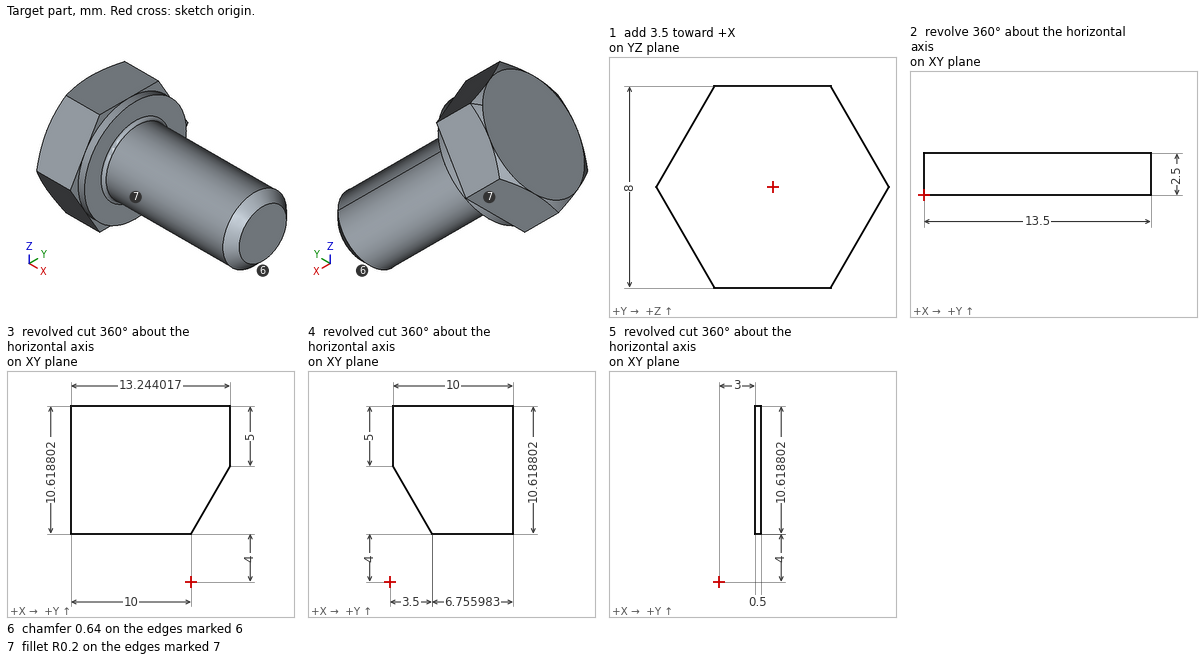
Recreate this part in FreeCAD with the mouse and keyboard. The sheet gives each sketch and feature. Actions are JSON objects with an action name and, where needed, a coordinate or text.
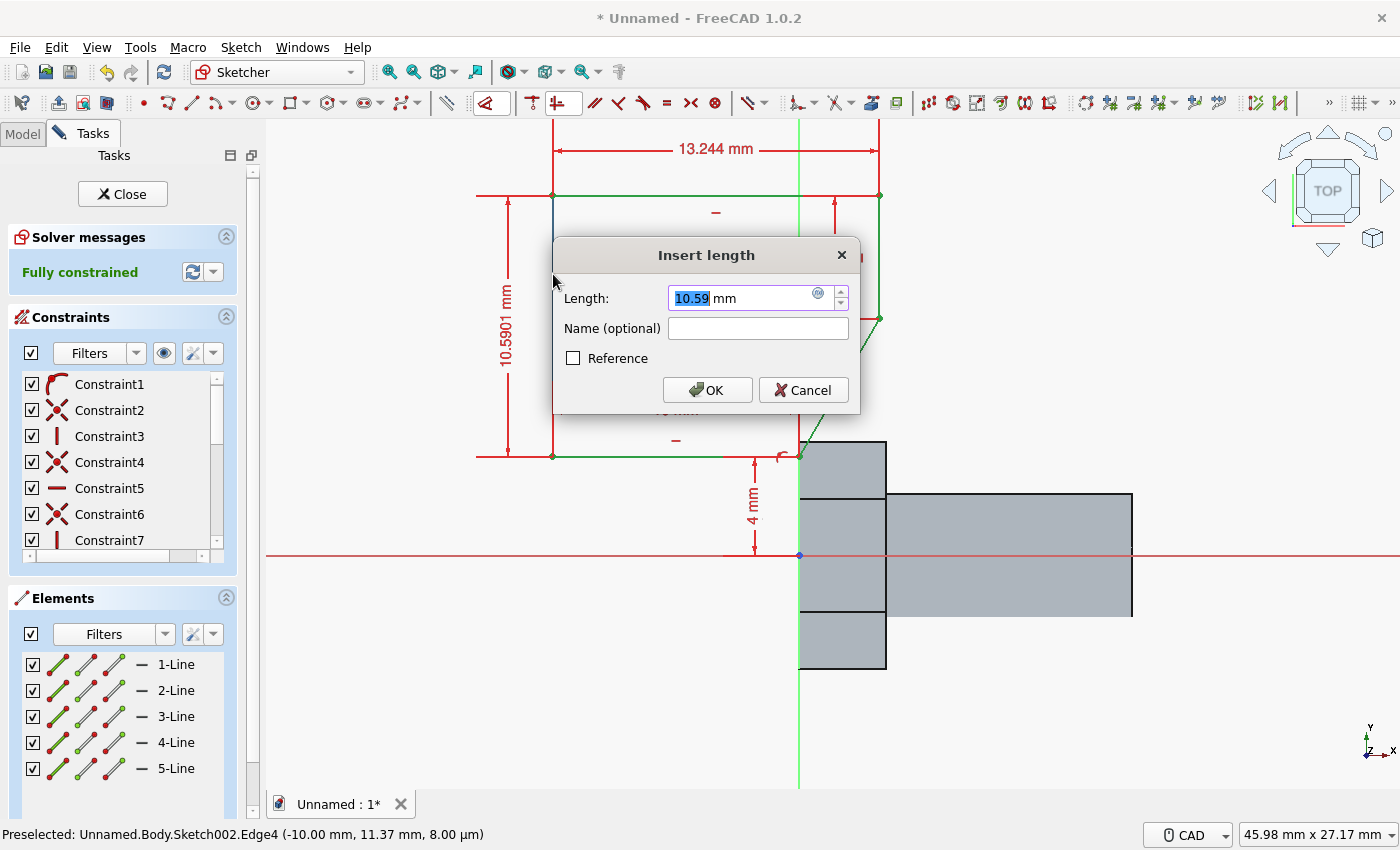
{"action": "type", "text": "10.618802"}
{"action": "key", "text": "Return"}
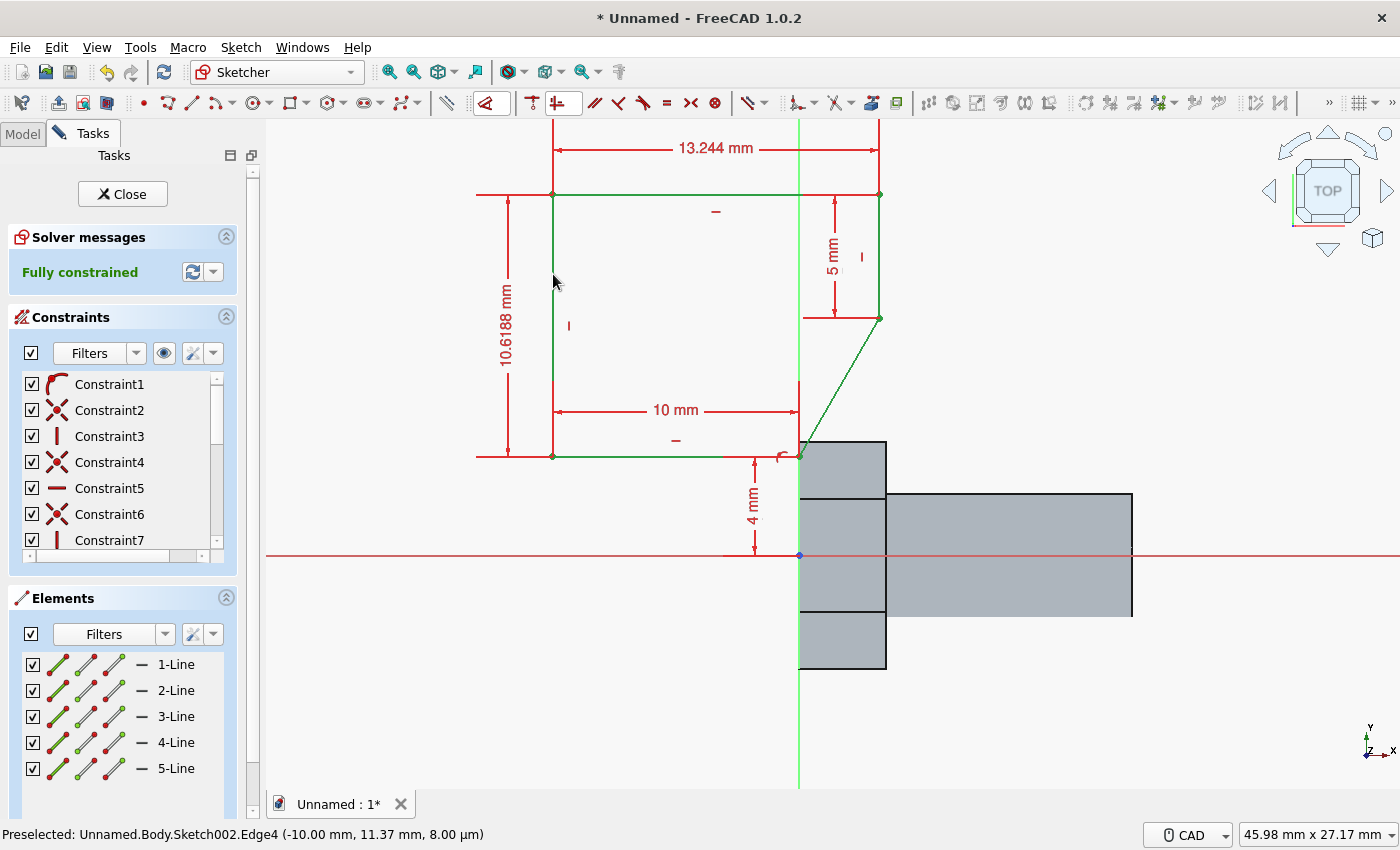
{"action": "left_click", "coordinate": [123, 194]}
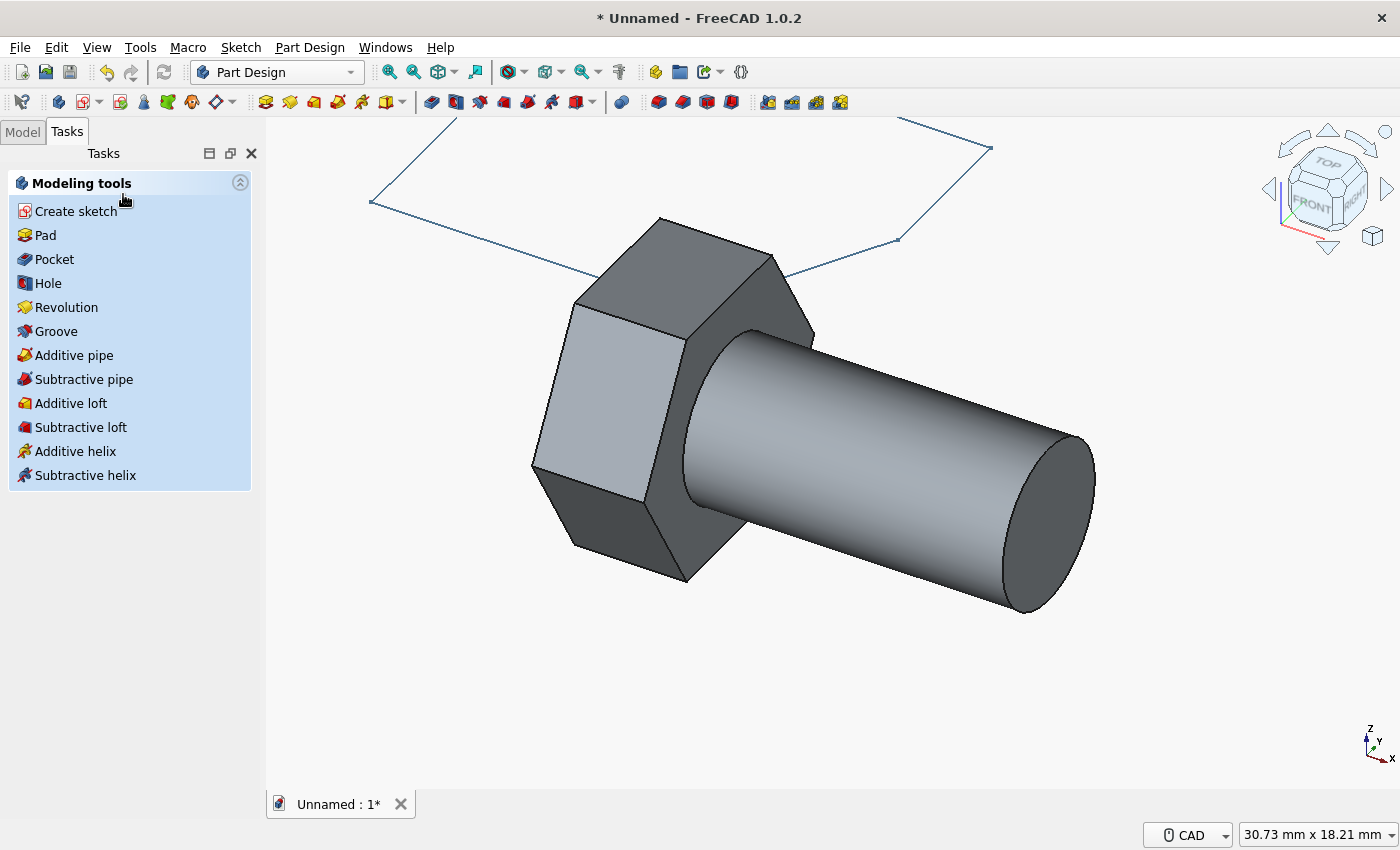
{"action": "left_click", "coordinate": [480, 102]}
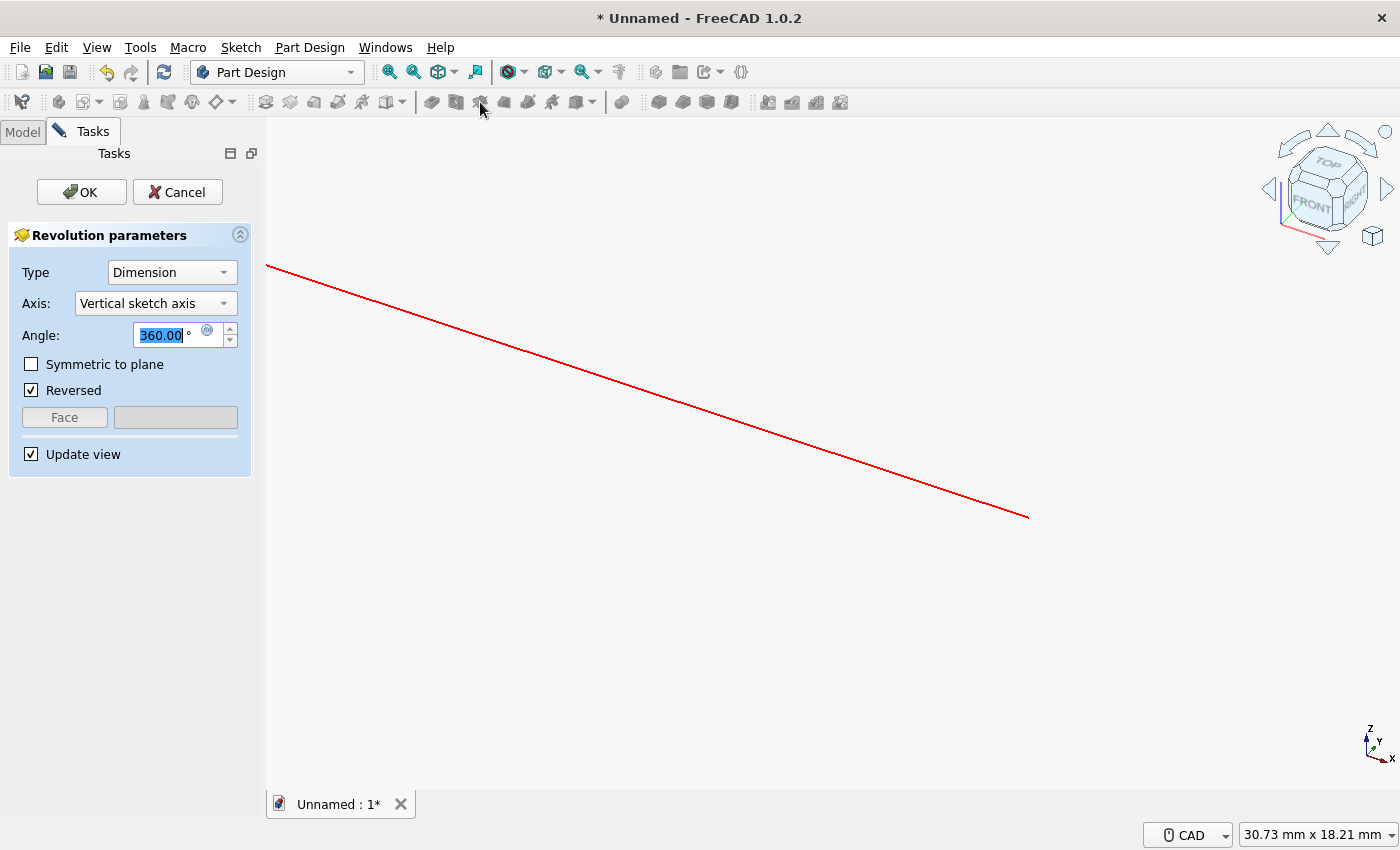
{"action": "left_click", "coordinate": [156, 304]}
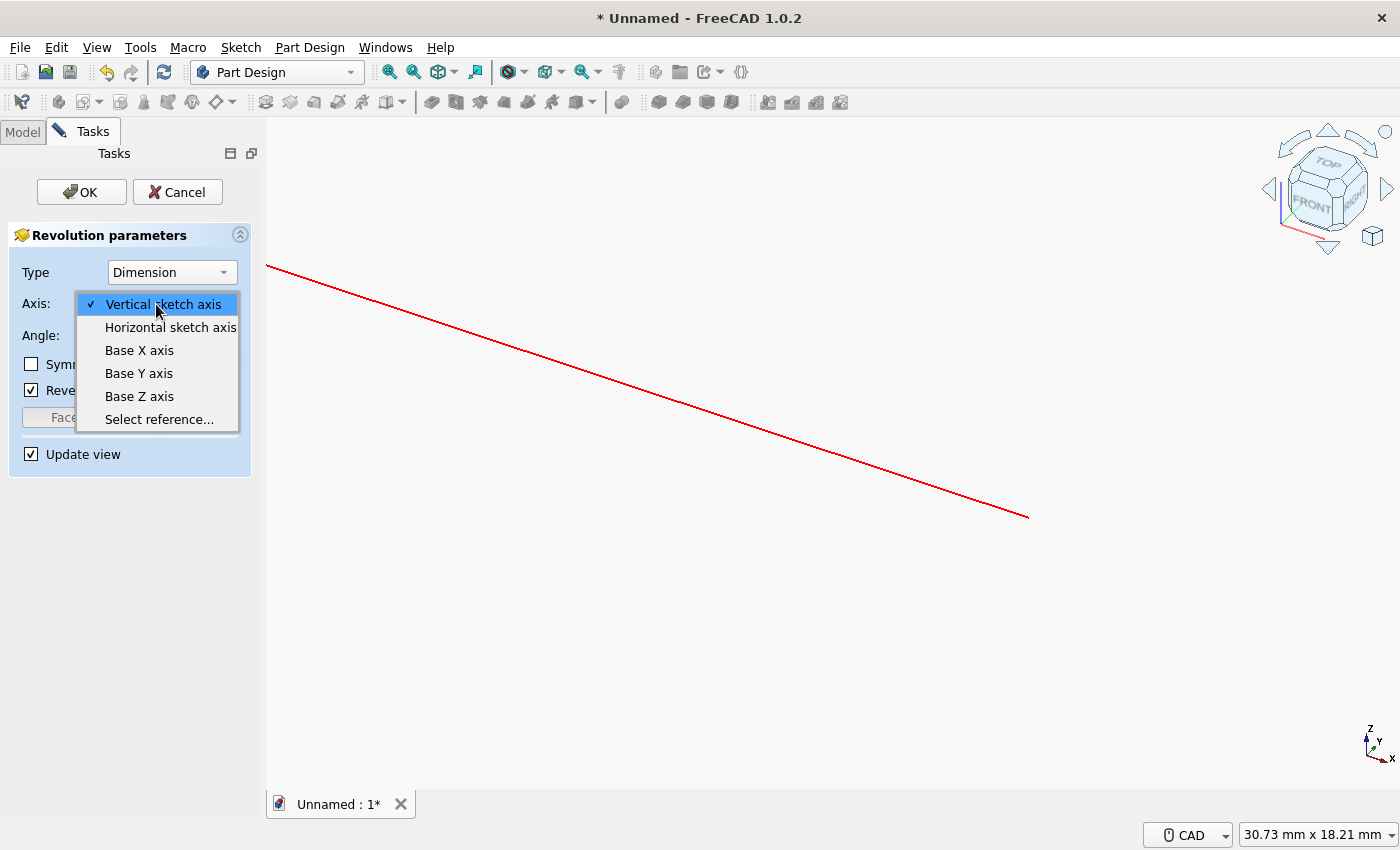
{"action": "left_click", "coordinate": [156, 328]}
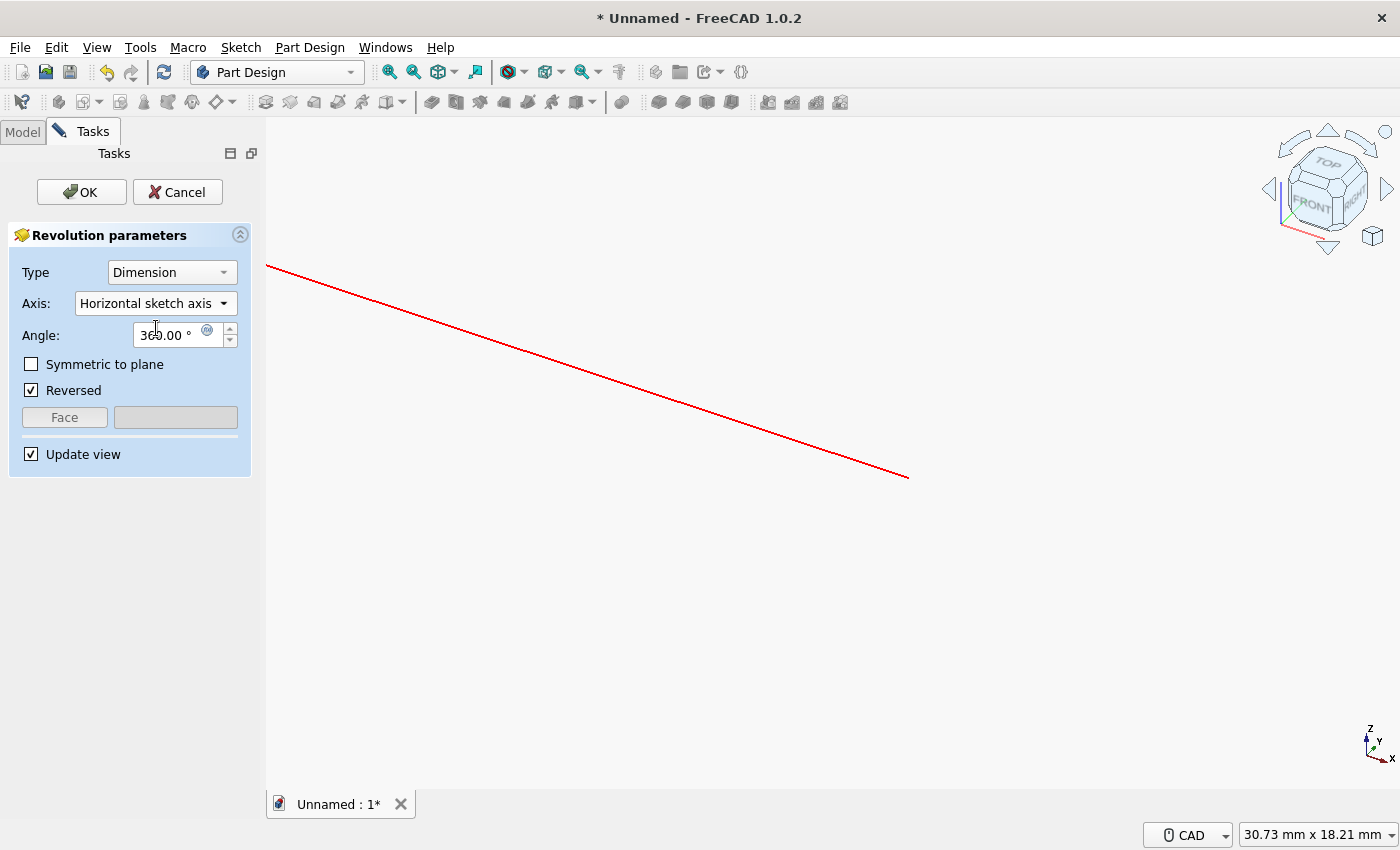
{"action": "left_click", "coordinate": [82, 192]}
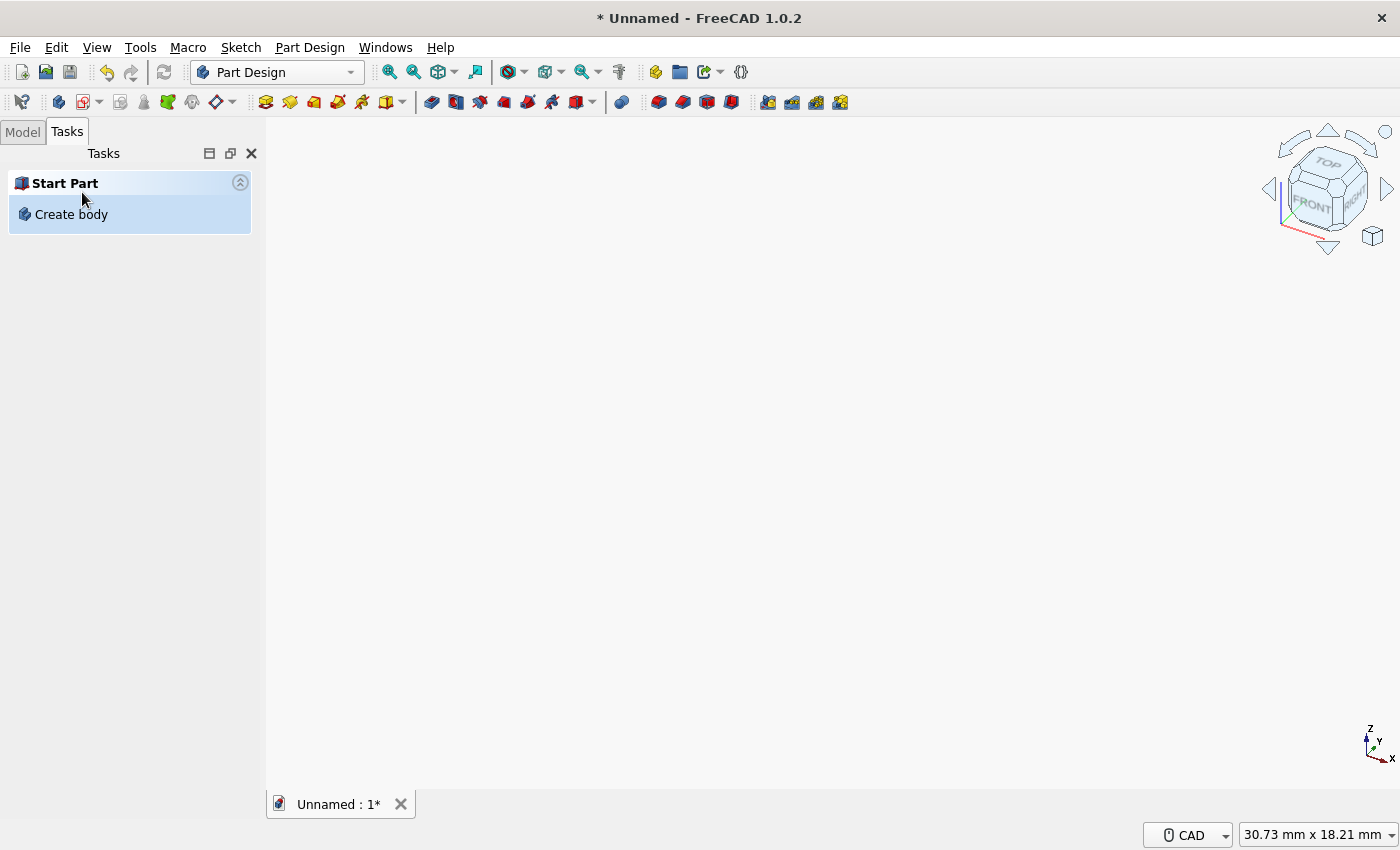
{"action": "left_click", "coordinate": [390, 72]}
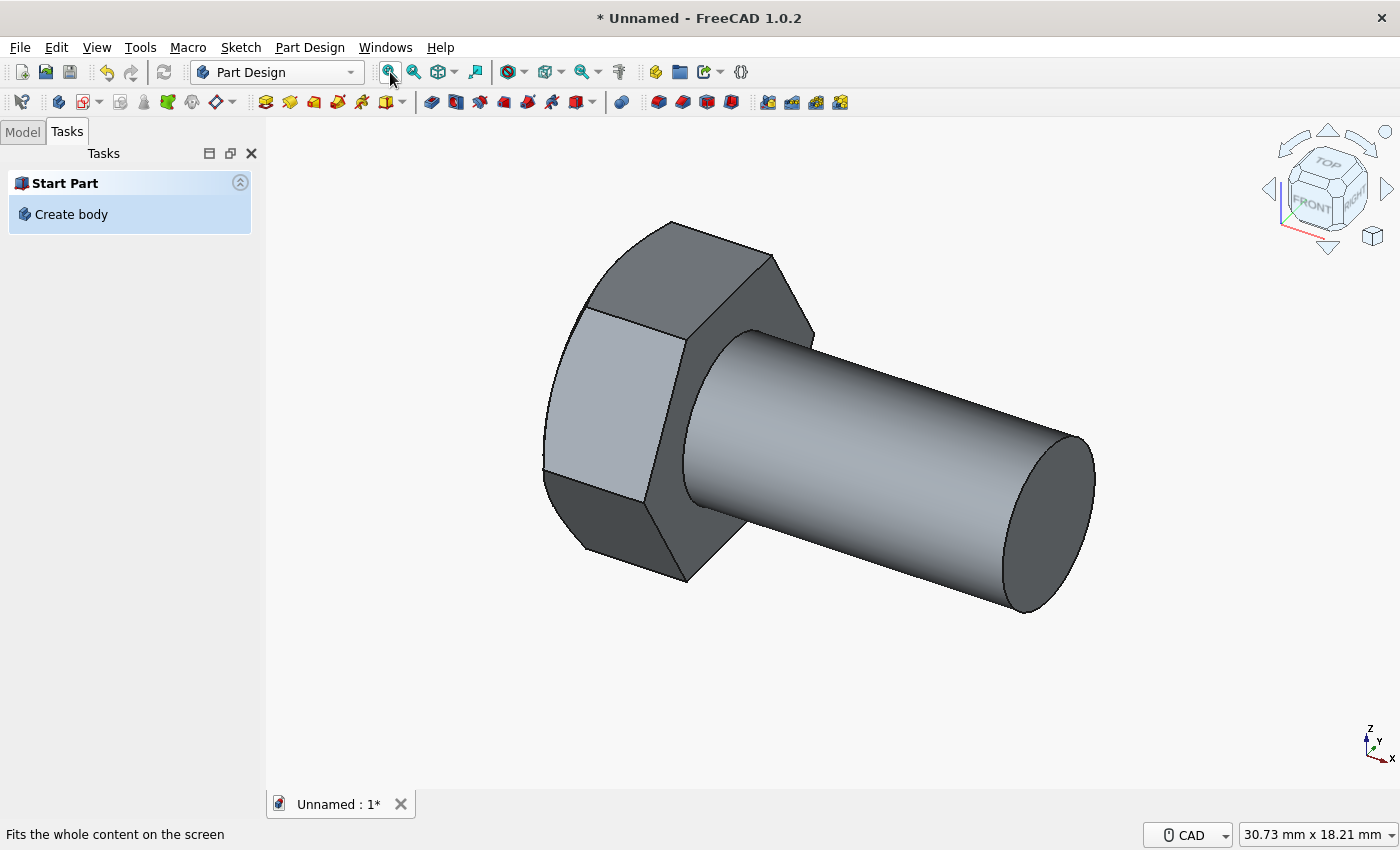
{"action": "left_click", "coordinate": [84, 102]}